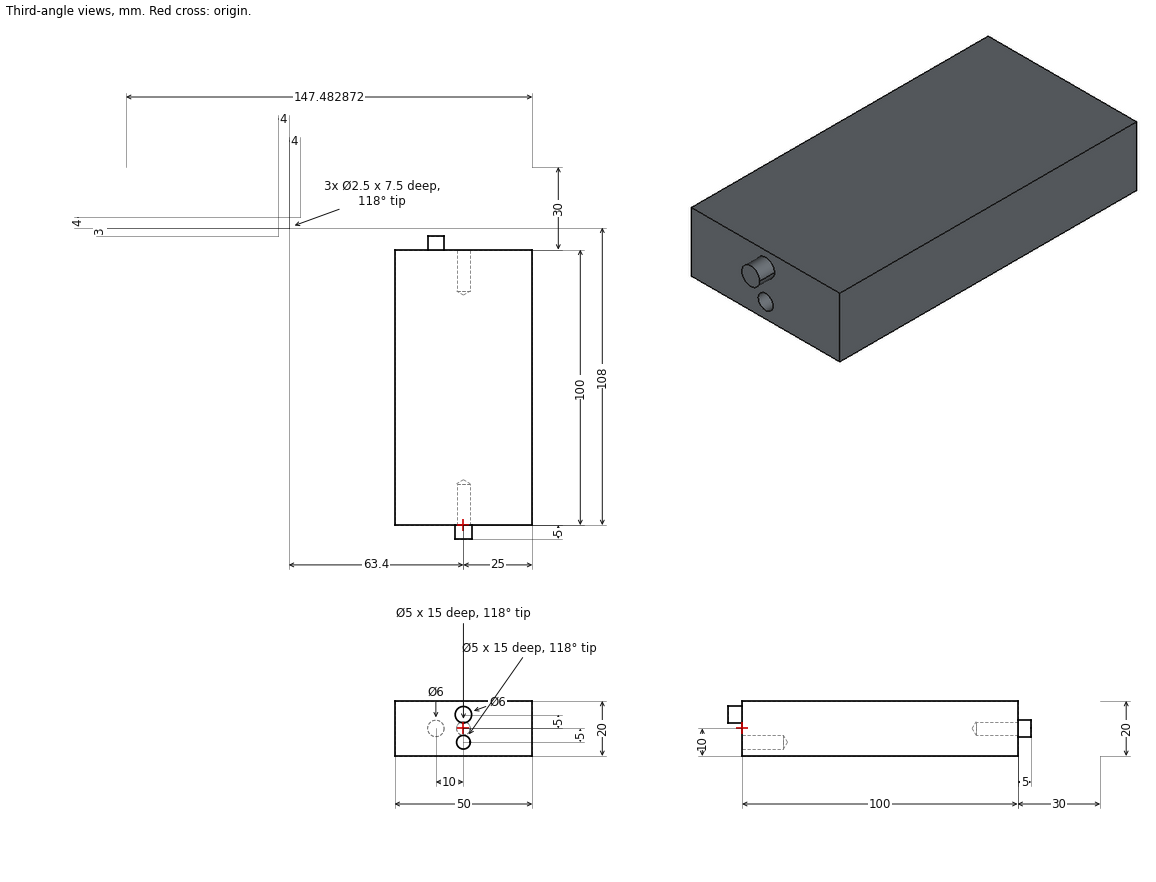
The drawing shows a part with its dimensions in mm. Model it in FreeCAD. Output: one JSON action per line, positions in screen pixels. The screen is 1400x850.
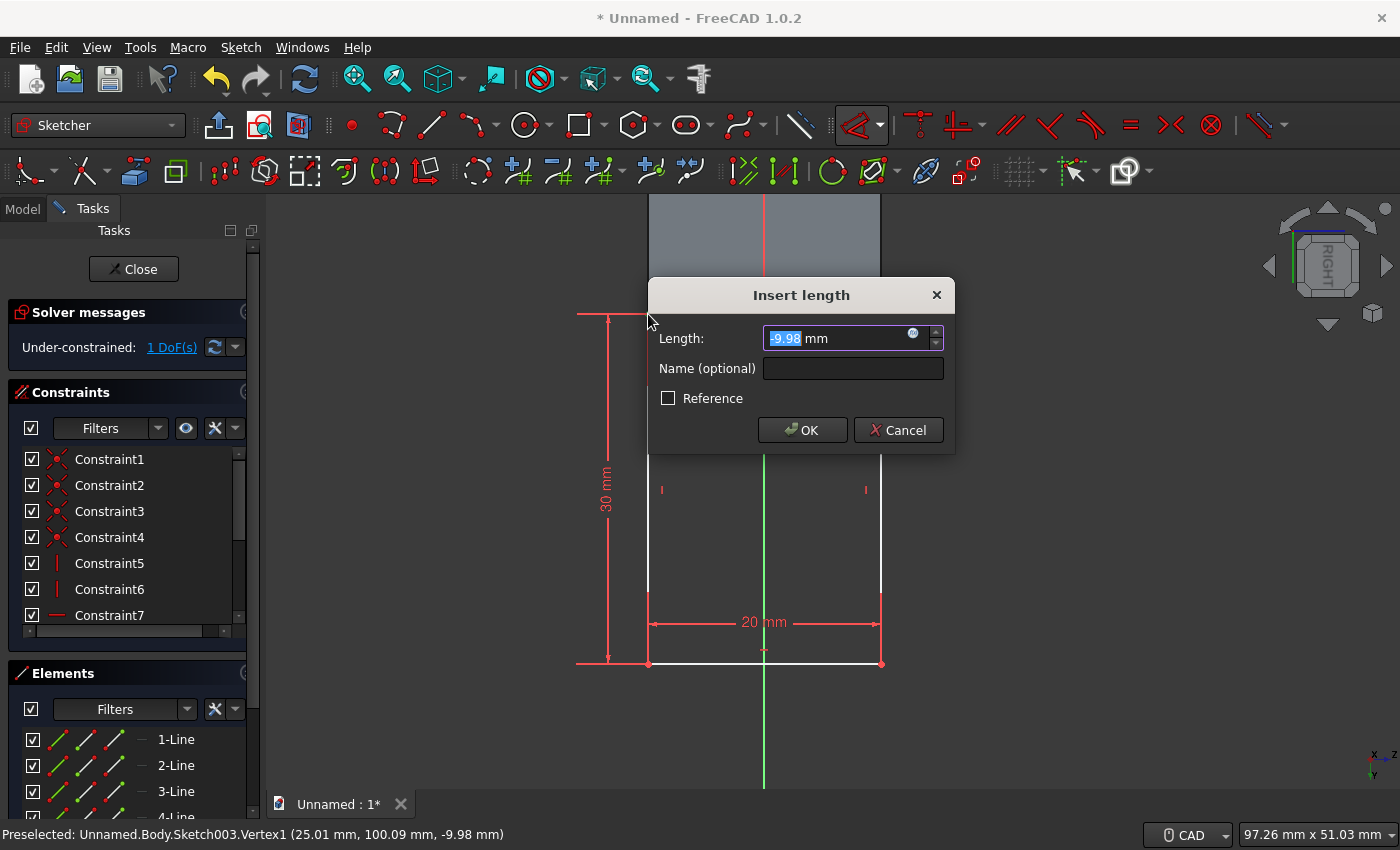
{"action": "type", "text": "-10"}
{"action": "key", "text": "Return"}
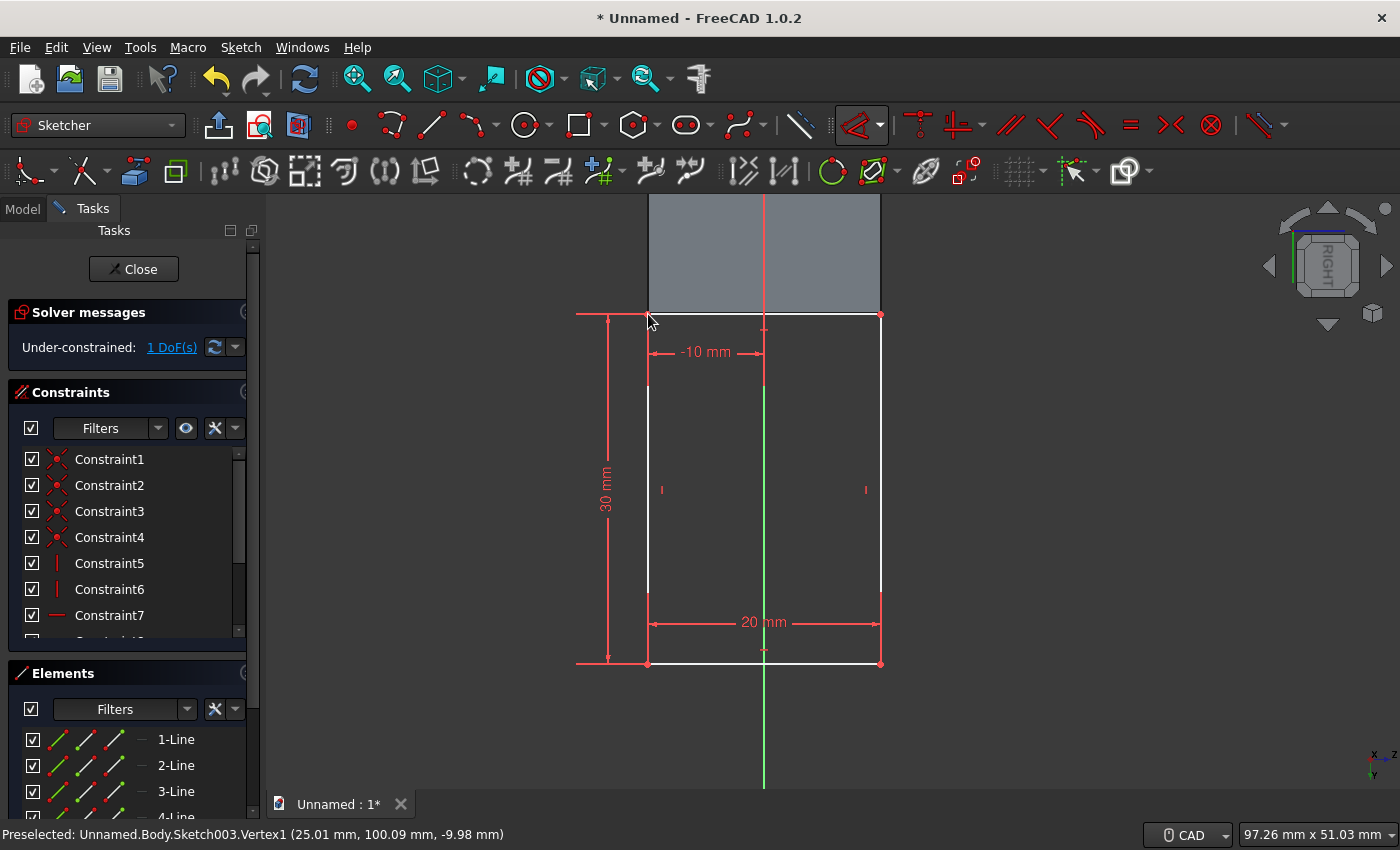
{"action": "left_click", "coordinate": [648, 314]}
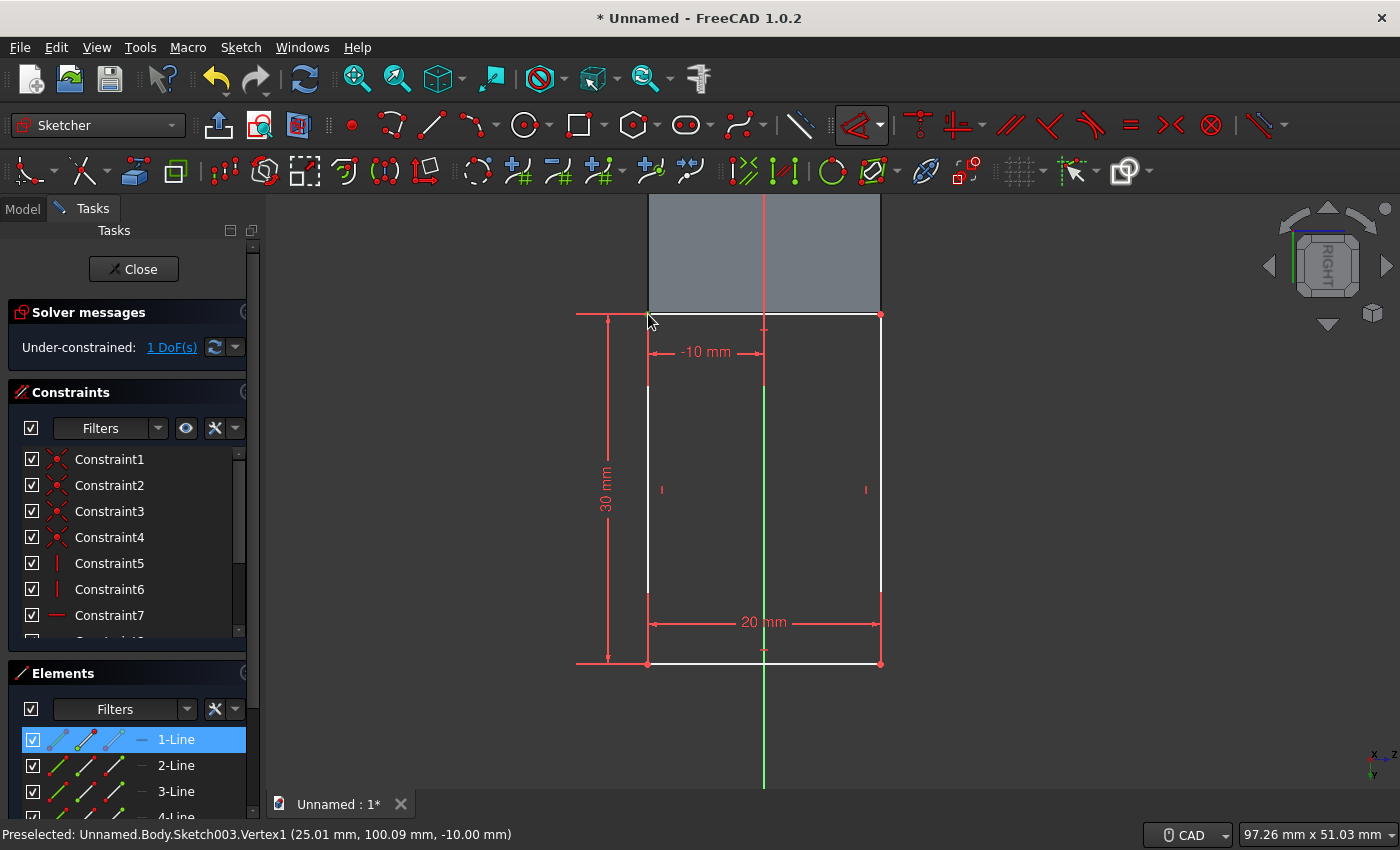
{"action": "key", "text": "i"}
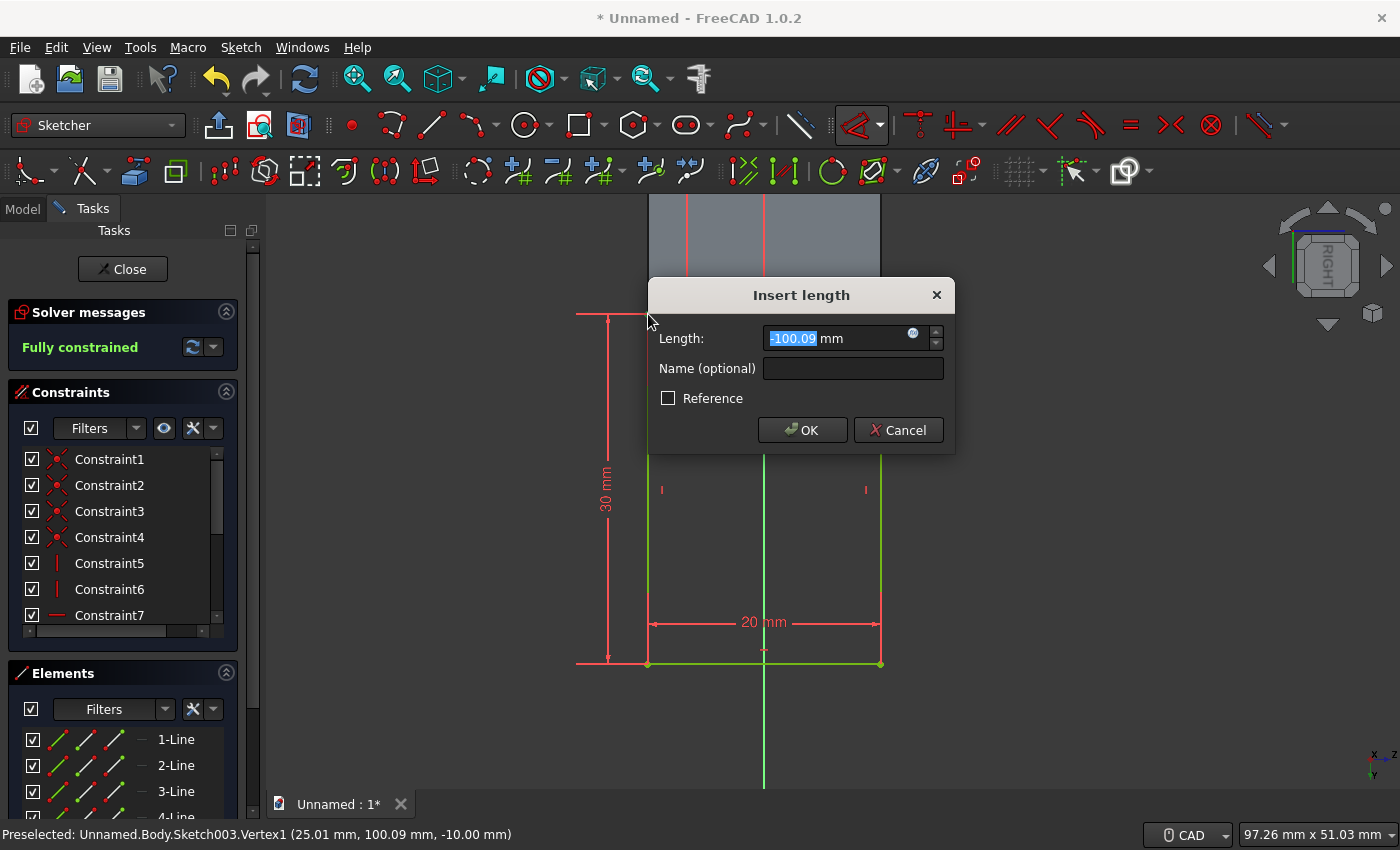
{"action": "type", "text": "-100"}
{"action": "key", "text": "Return"}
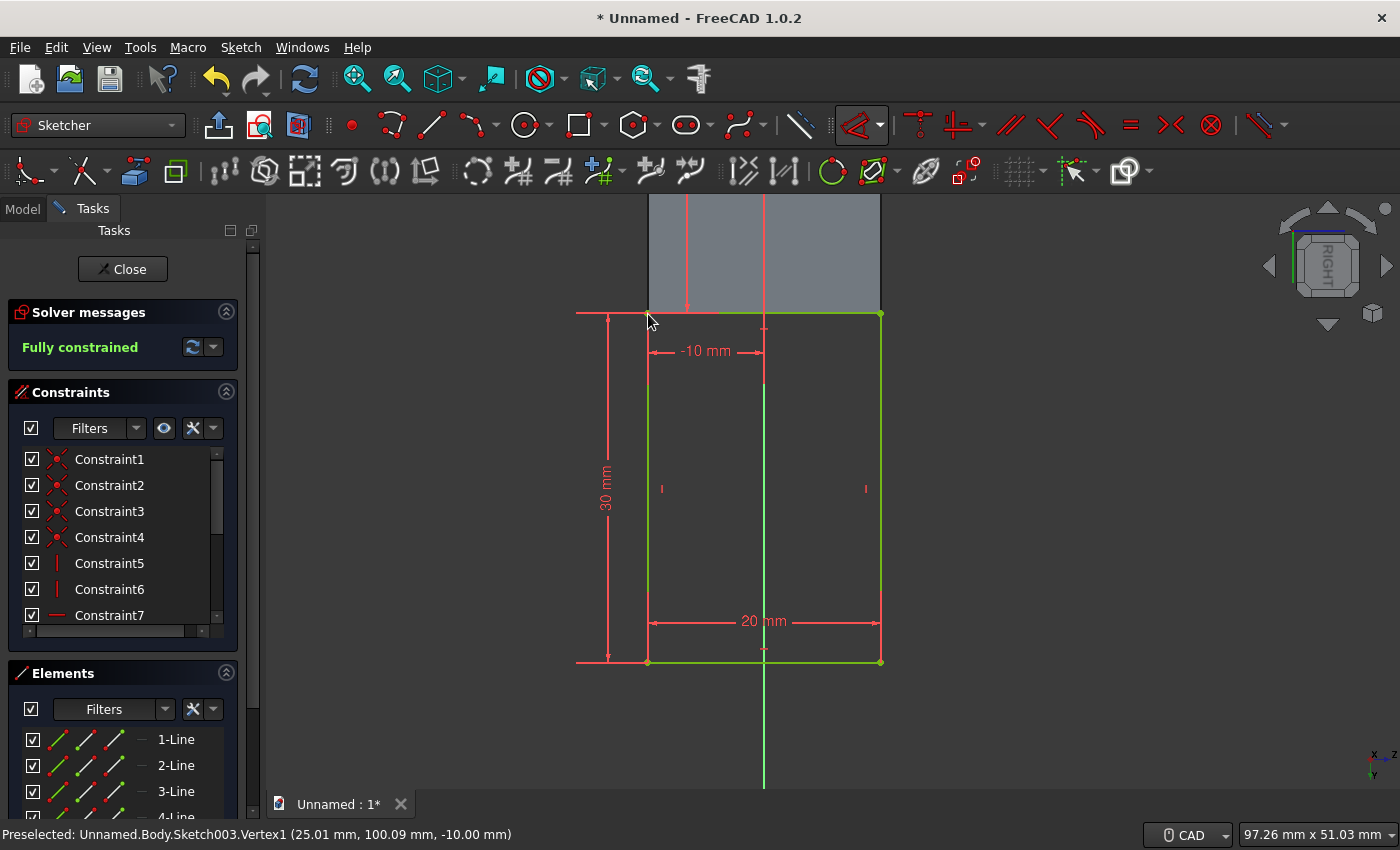
{"action": "left_click", "coordinate": [123, 269]}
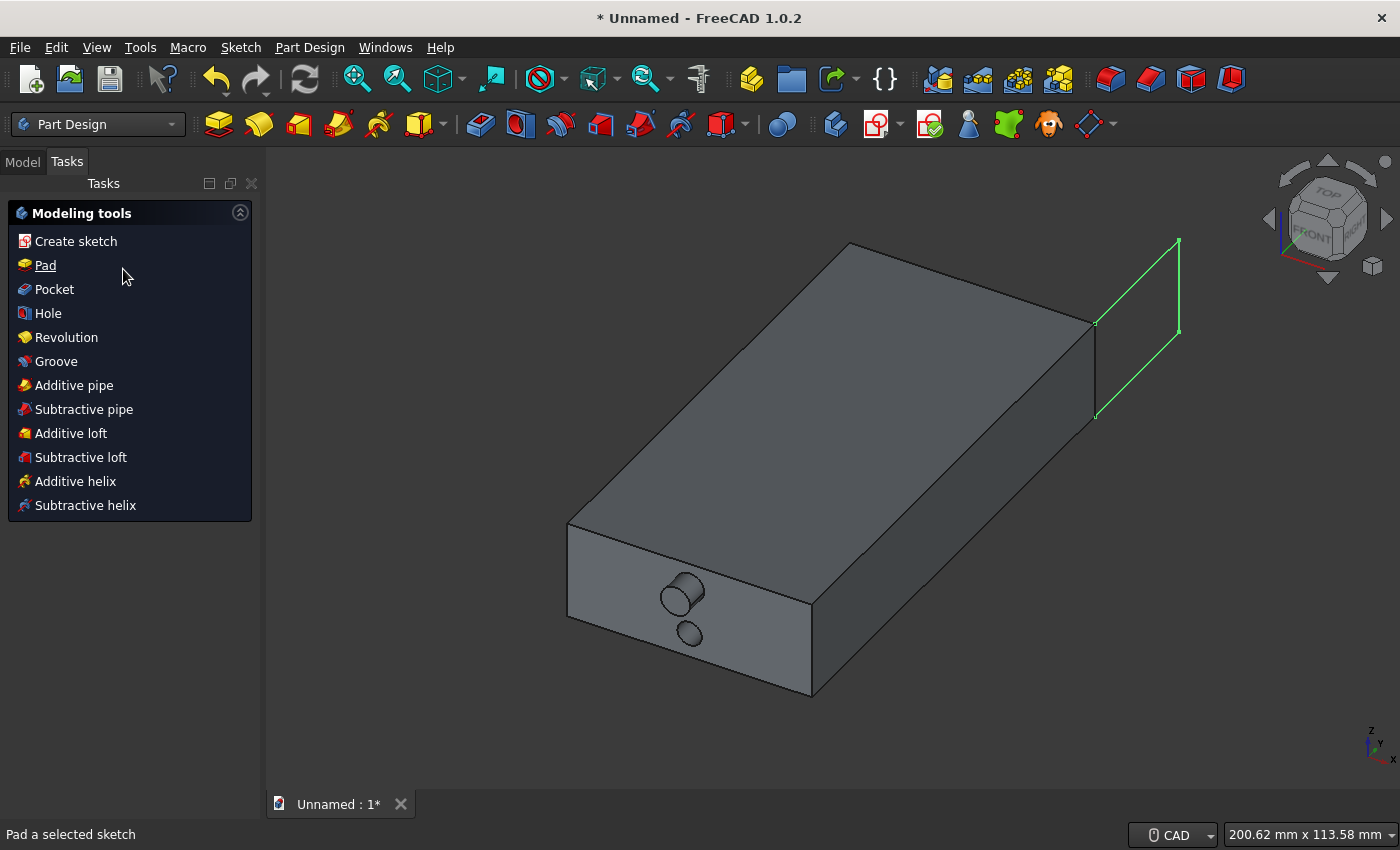
{"action": "left_click", "coordinate": [220, 124]}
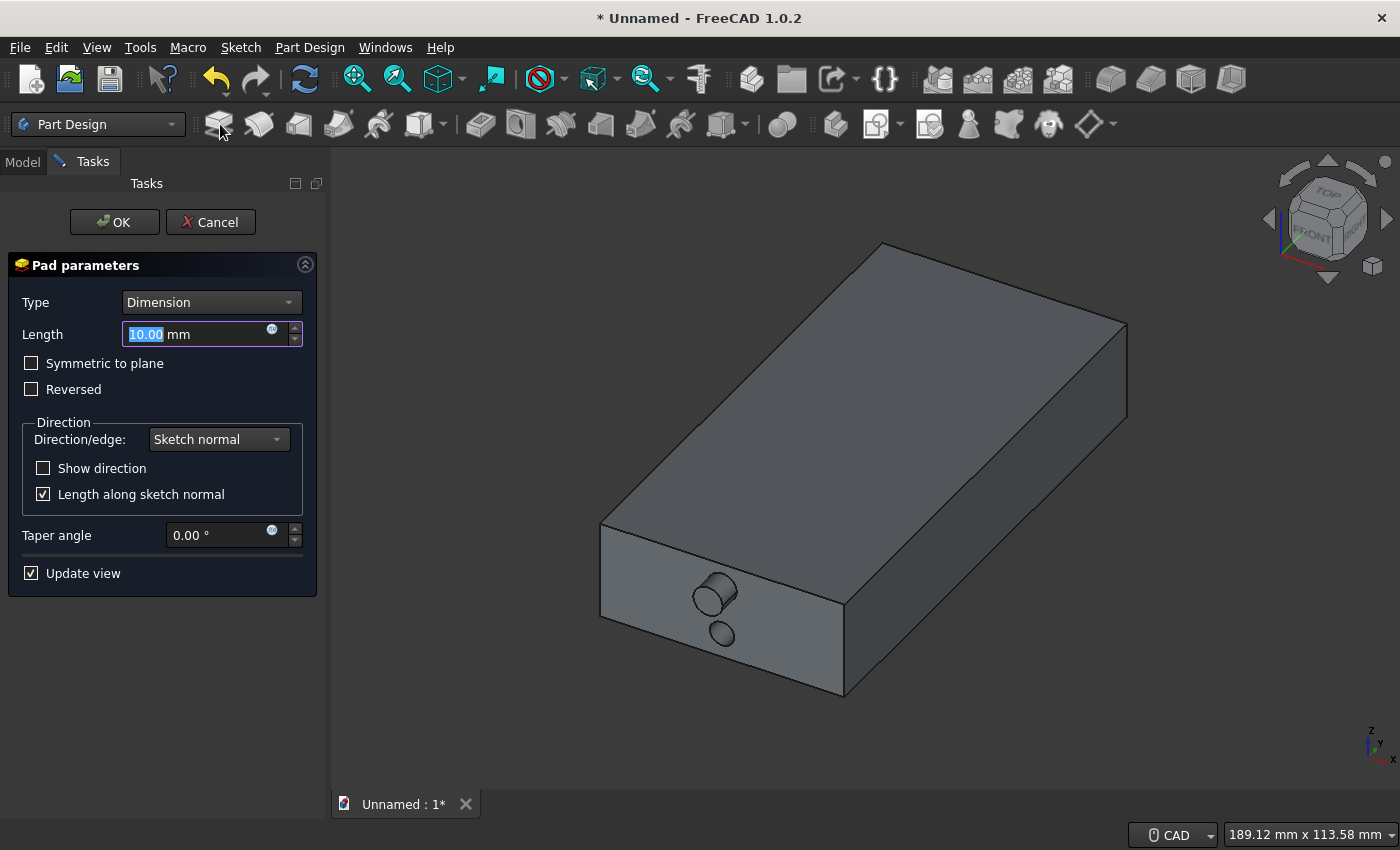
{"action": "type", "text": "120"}
{"action": "key", "text": "Tab"}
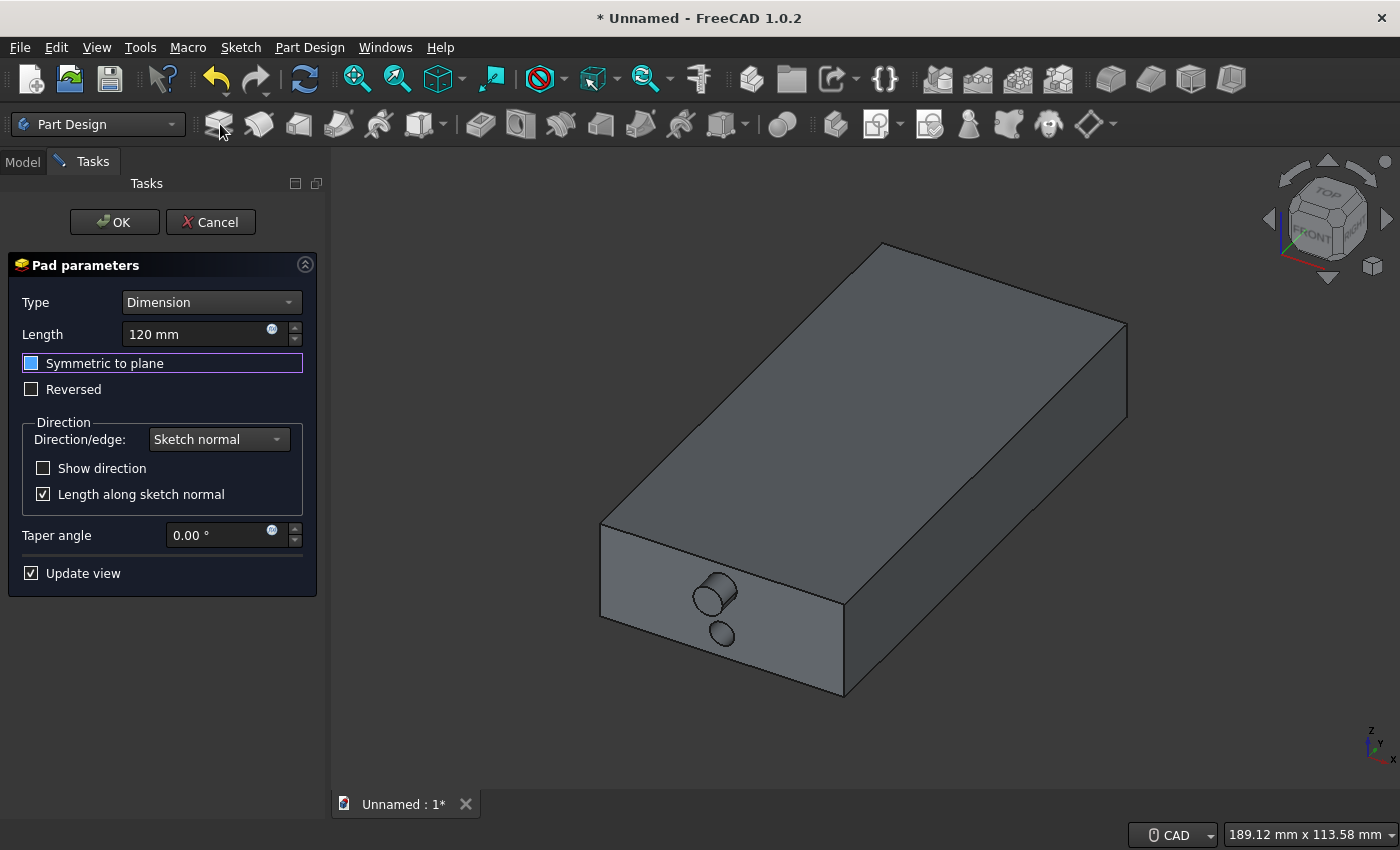
{"action": "left_click", "coordinate": [30, 389]}